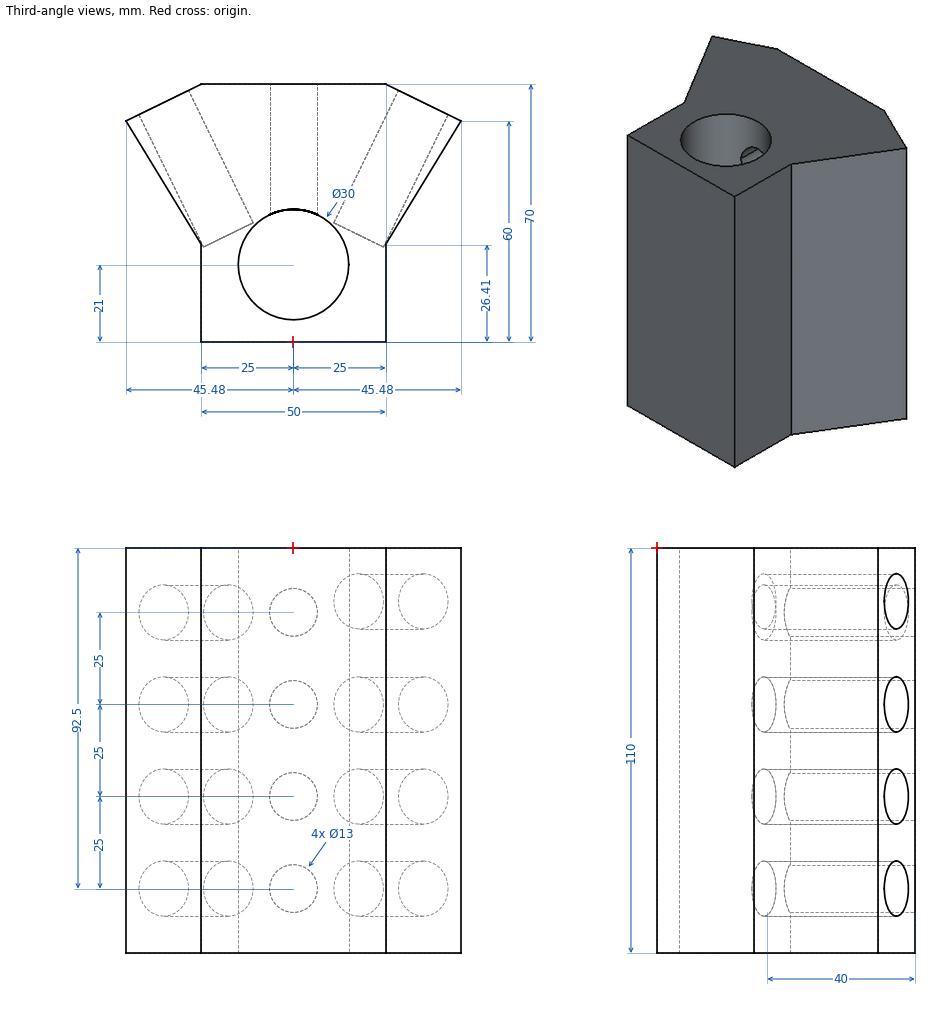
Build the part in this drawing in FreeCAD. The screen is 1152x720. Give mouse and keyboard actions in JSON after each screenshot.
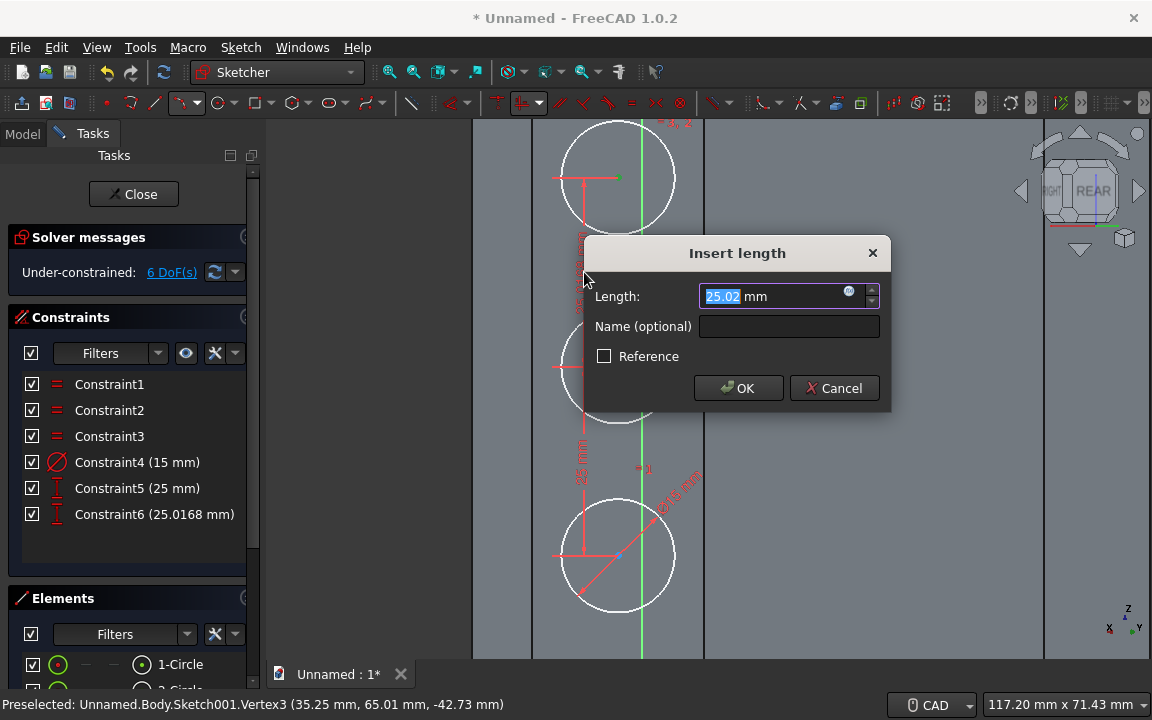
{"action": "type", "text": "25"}
{"action": "key", "text": "Return"}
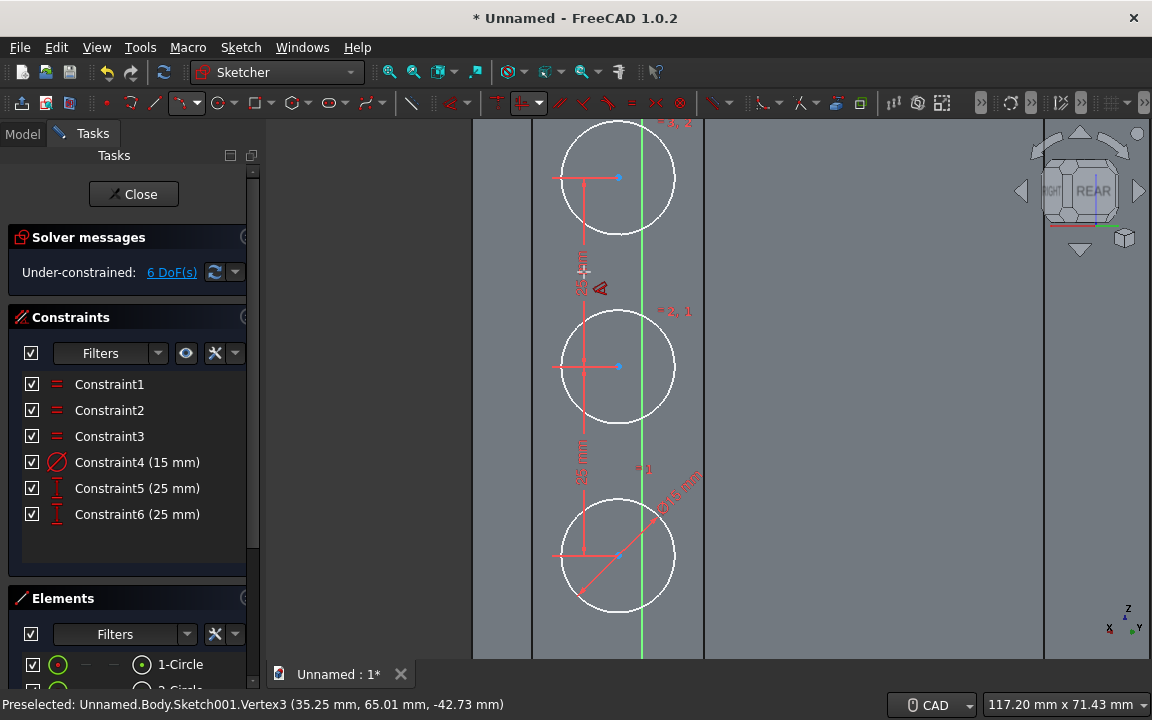
{"action": "left_click", "coordinate": [618, 178]}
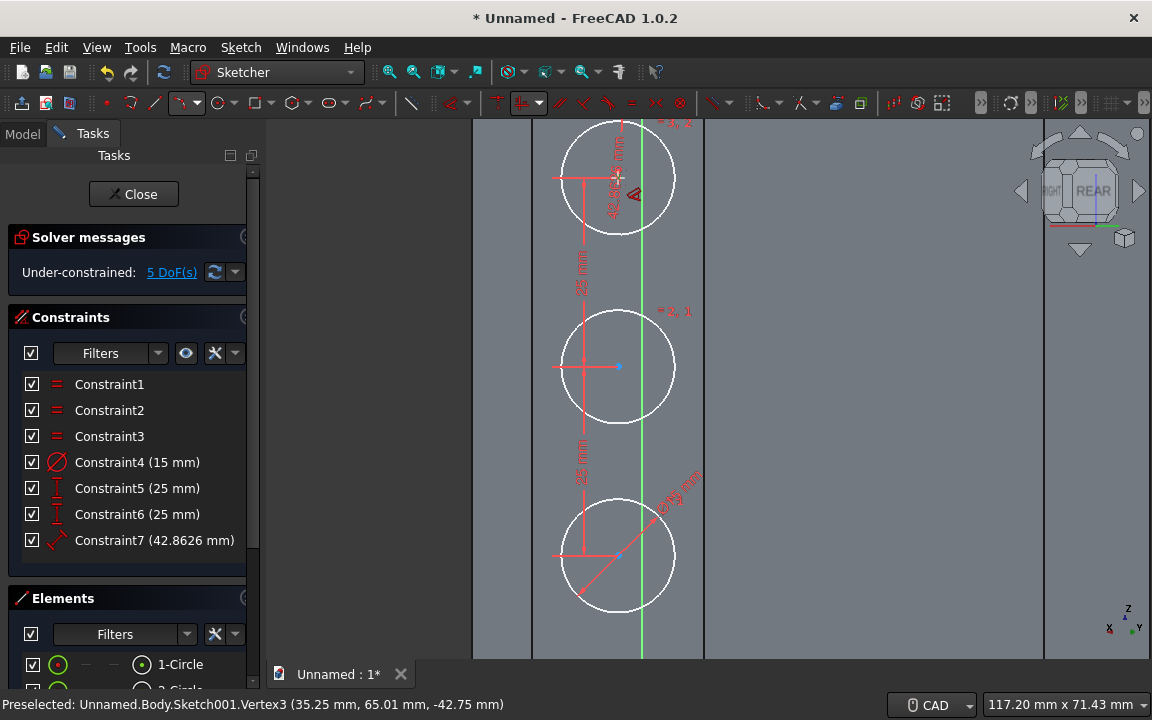
{"action": "scroll", "coordinate": [659, 517], "scroll_direction": "down", "scroll_amount": 4}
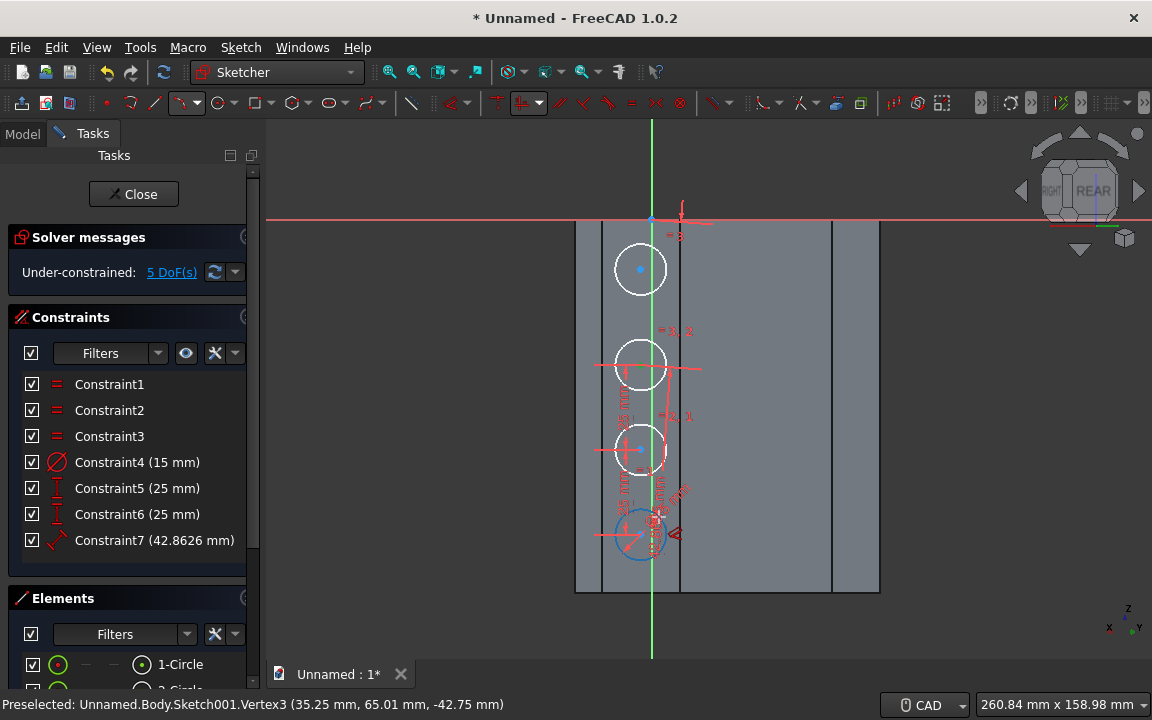
{"action": "left_click", "coordinate": [641, 270]}
{"action": "left_click", "coordinate": [607, 317]}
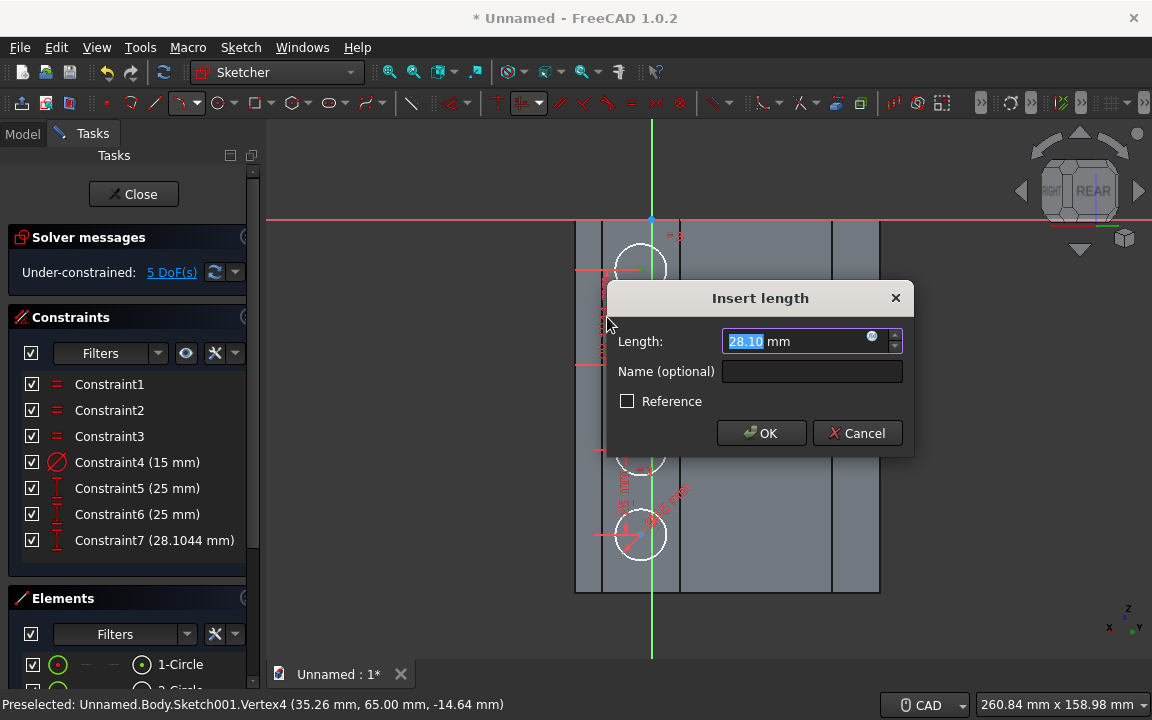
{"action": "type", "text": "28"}
{"action": "key", "text": "Return"}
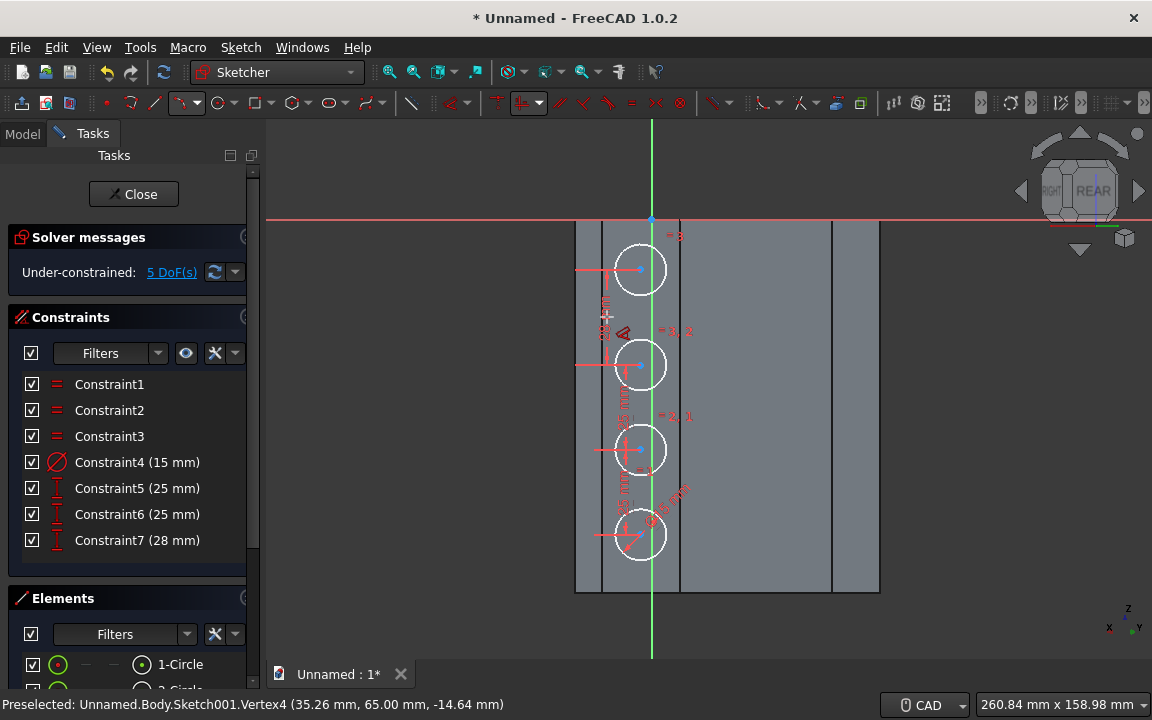
{"action": "left_click", "coordinate": [641, 535]}
{"action": "left_click", "coordinate": [686, 377]}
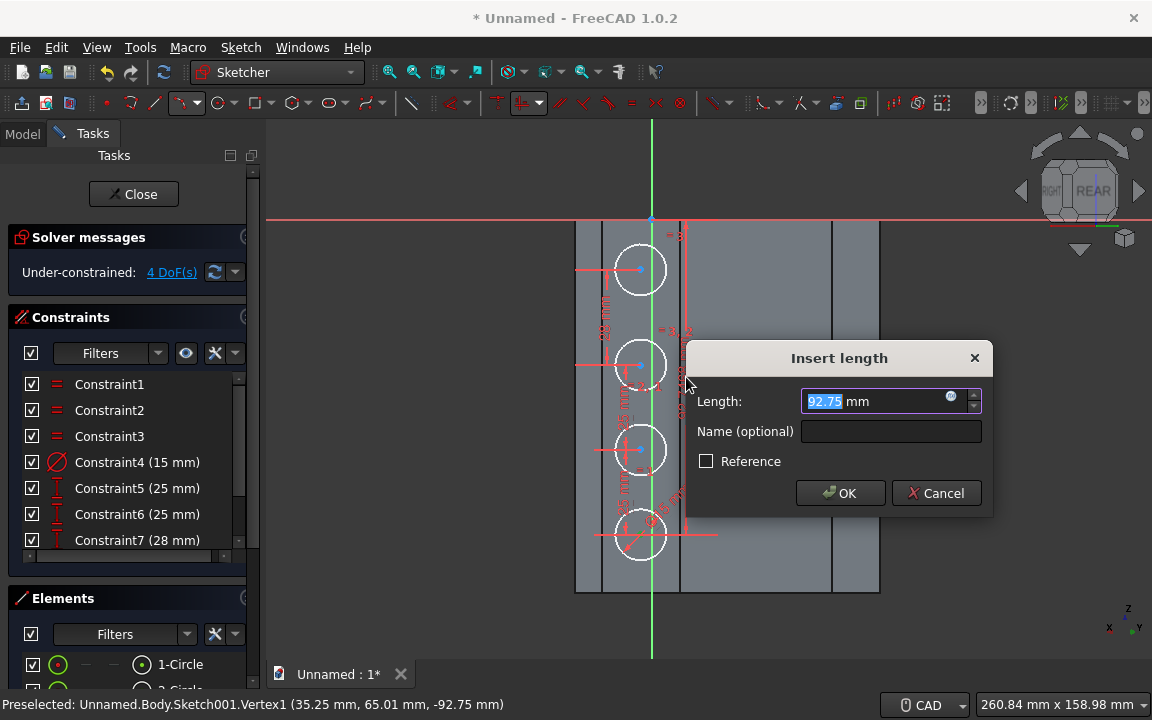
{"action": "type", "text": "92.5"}
{"action": "key", "text": "Return"}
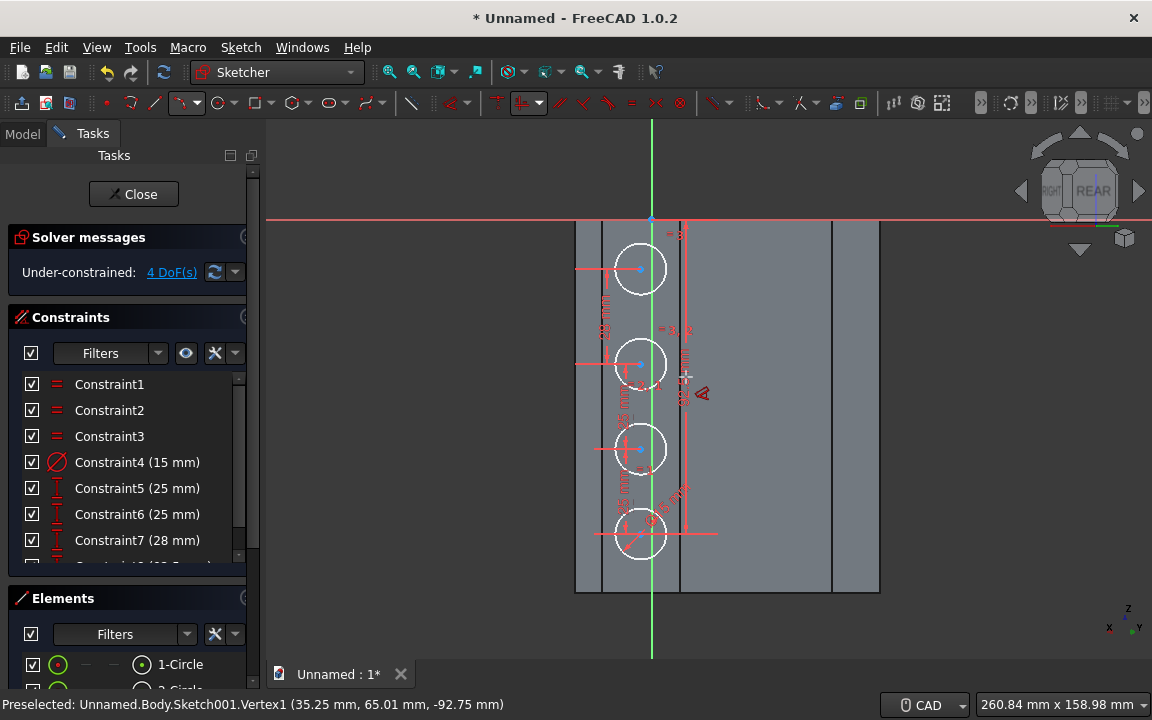
{"action": "scroll", "coordinate": [641, 534], "scroll_direction": "up", "scroll_amount": 7}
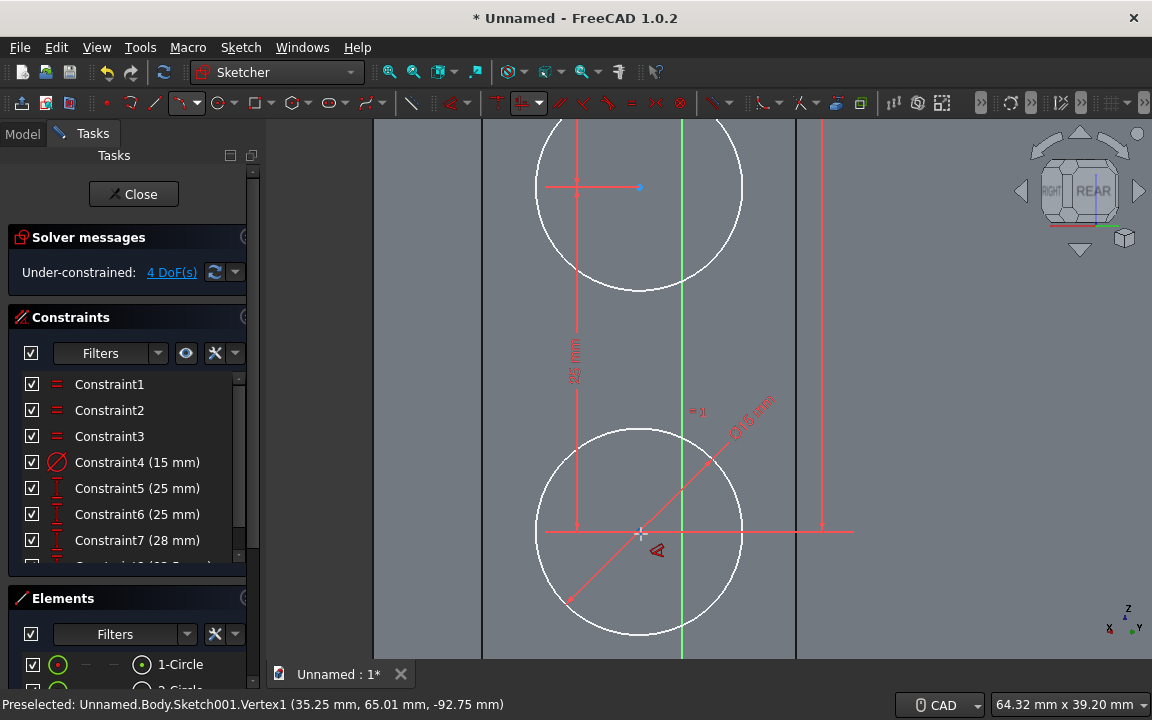
{"action": "left_click", "coordinate": [639, 532]}
{"action": "left_click", "coordinate": [661, 566]}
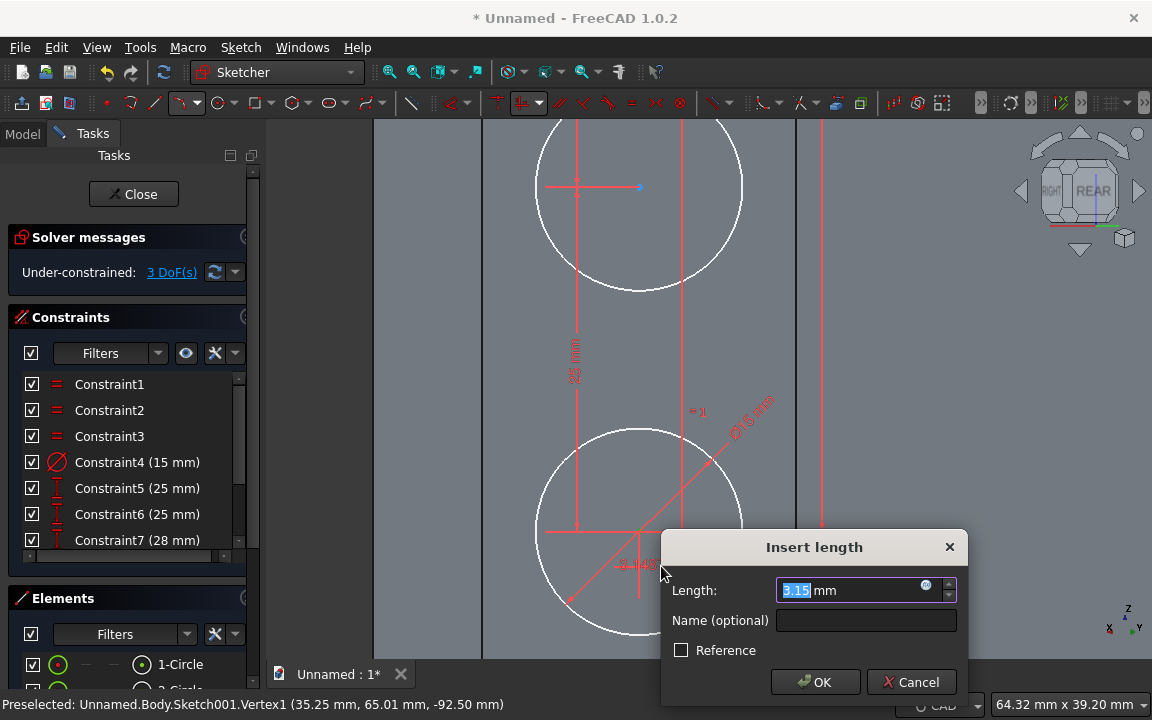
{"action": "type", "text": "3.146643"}
{"action": "key", "text": "Return"}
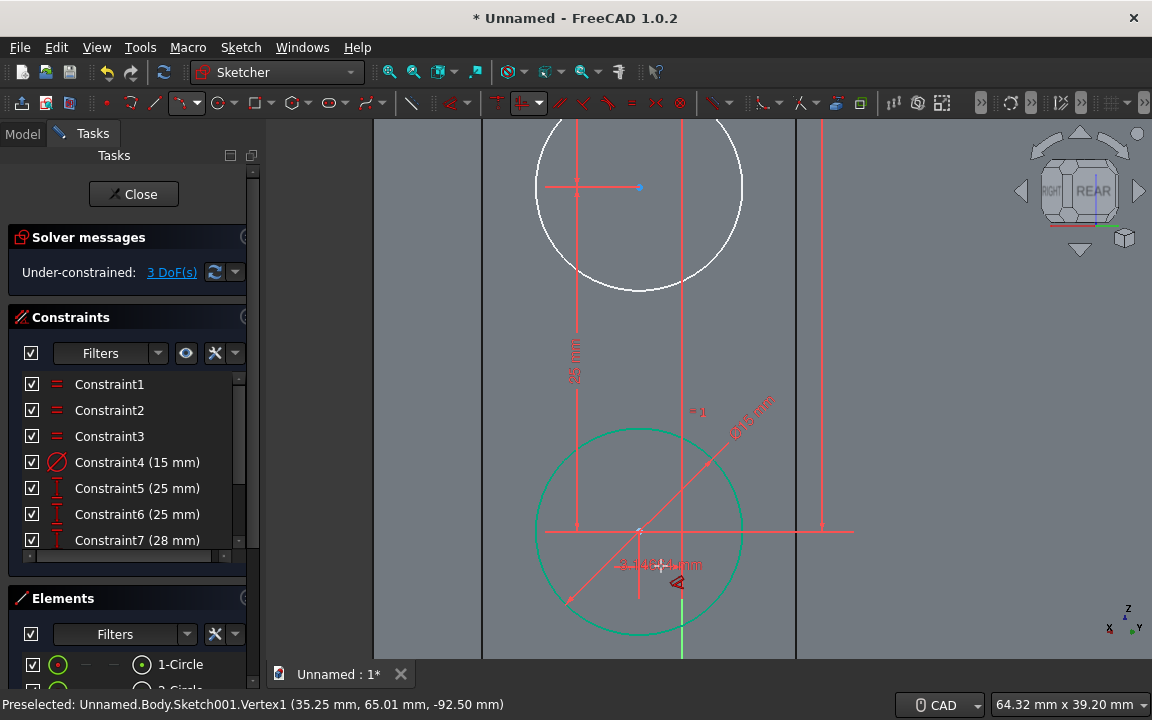
{"action": "left_click", "coordinate": [639, 187]}
{"action": "left_click", "coordinate": [661, 221]}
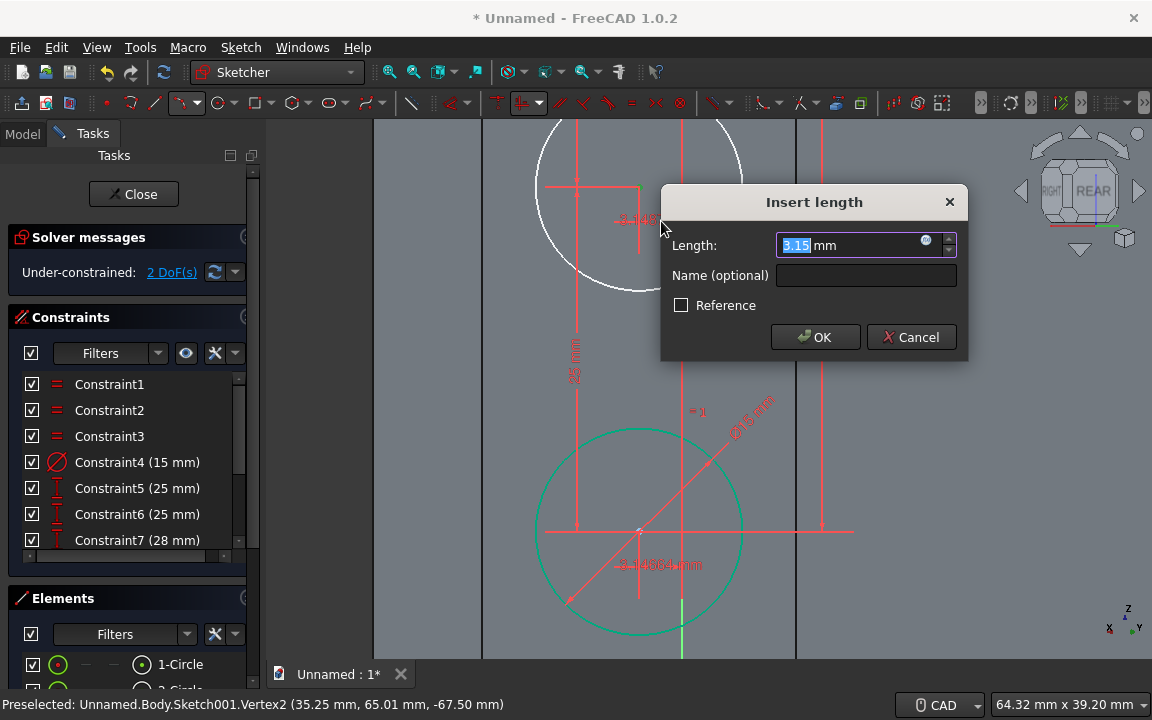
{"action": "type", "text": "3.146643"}
{"action": "key", "text": "Return"}